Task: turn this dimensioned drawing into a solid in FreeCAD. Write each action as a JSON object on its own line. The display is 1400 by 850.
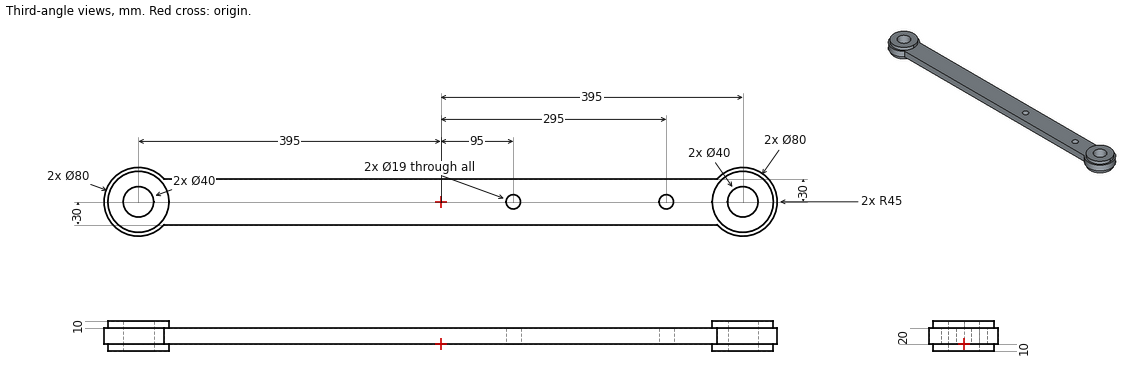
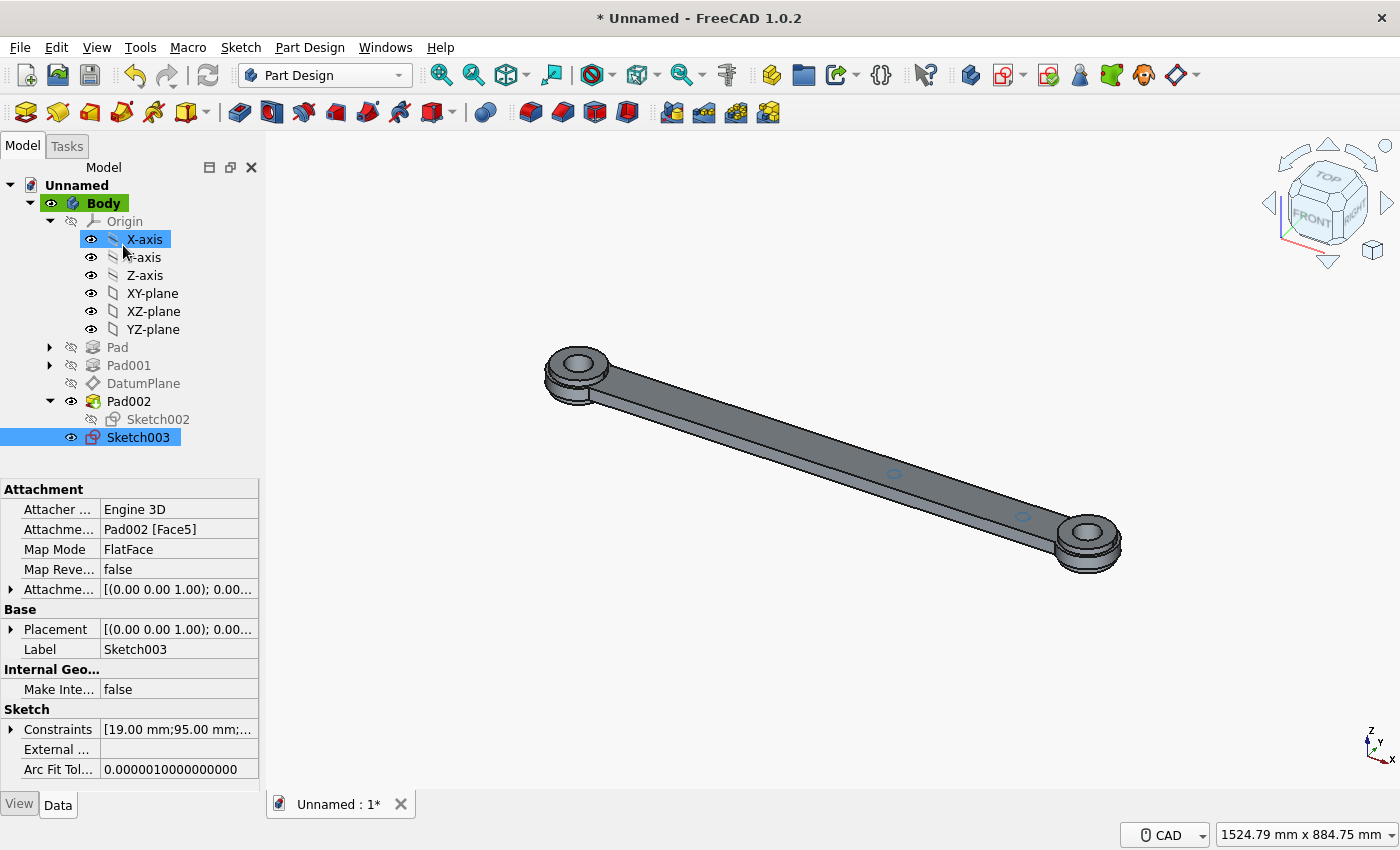
{"action": "left_click", "coordinate": [272, 112]}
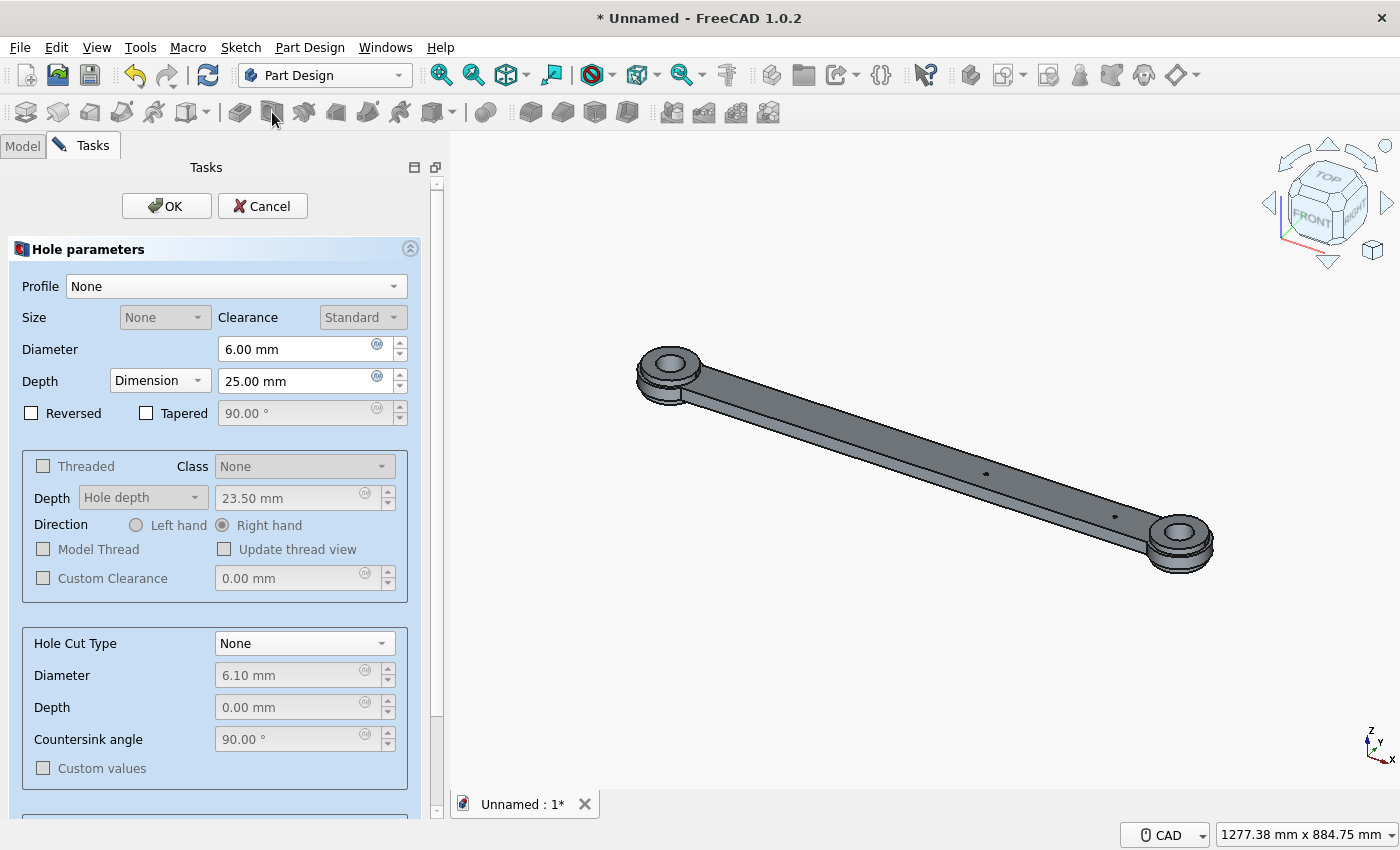
{"action": "triple_click", "coordinate": [305, 349]}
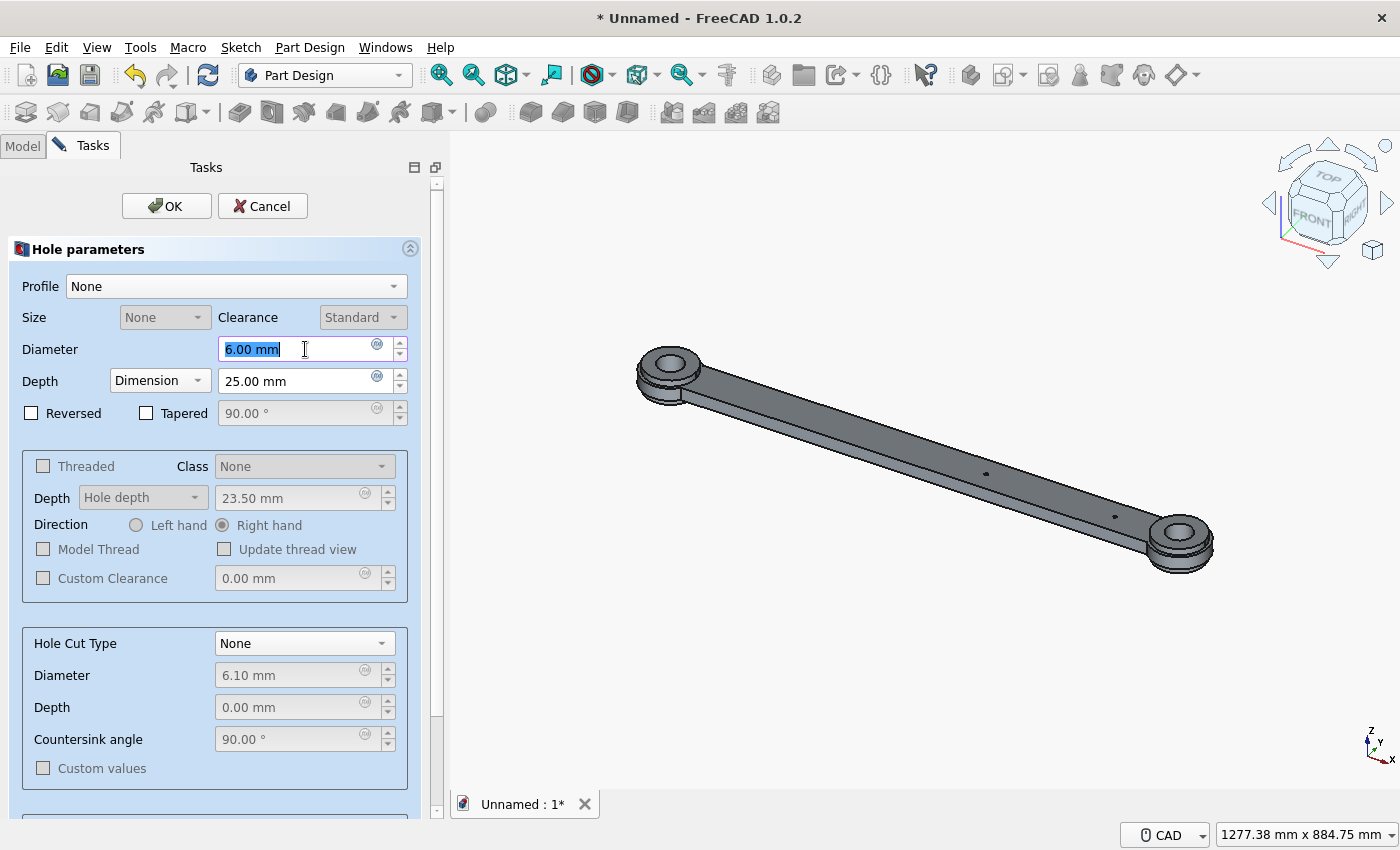
{"action": "type", "text": "19"}
{"action": "key", "text": "Tab"}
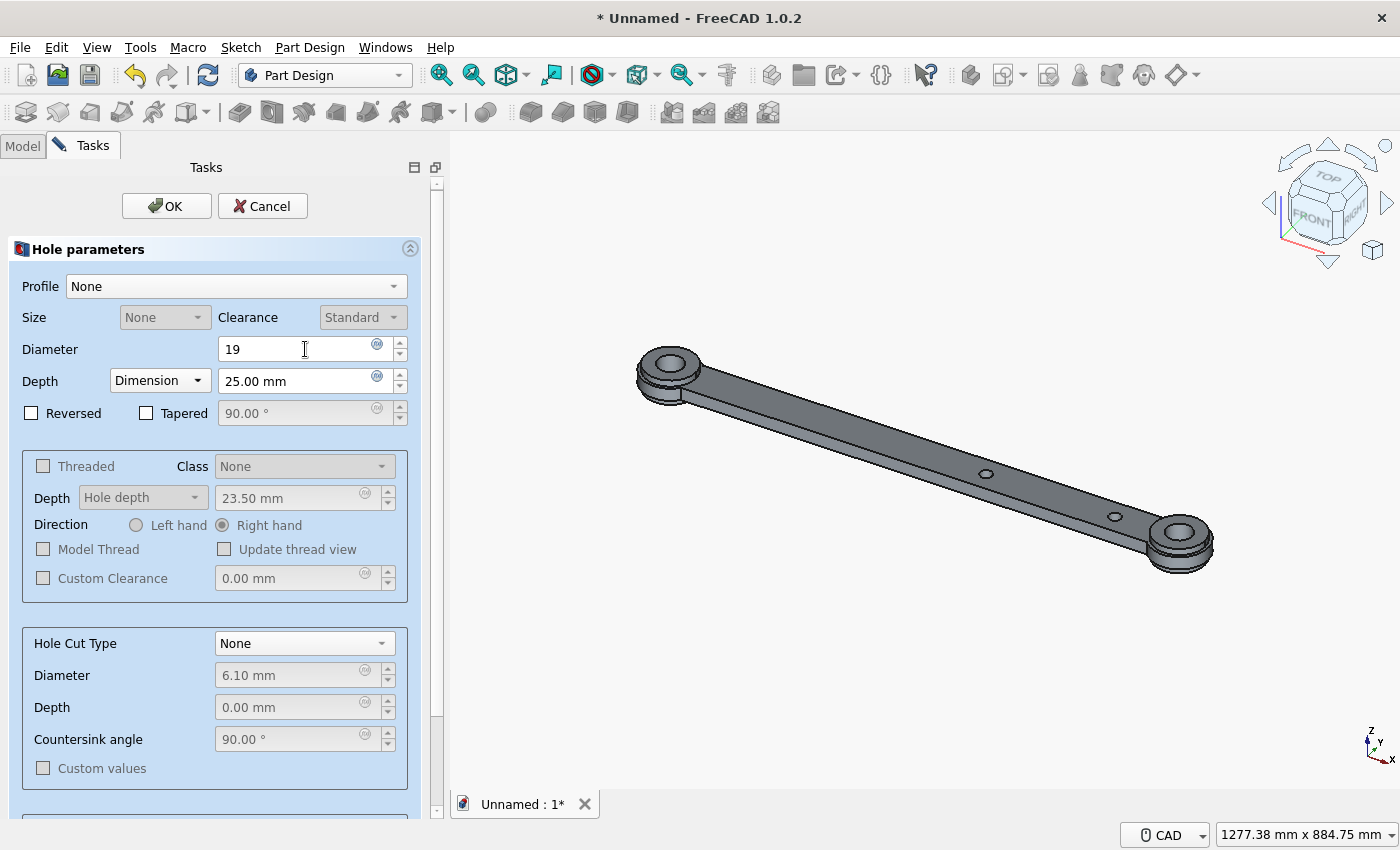
{"action": "left_click", "coordinate": [161, 380]}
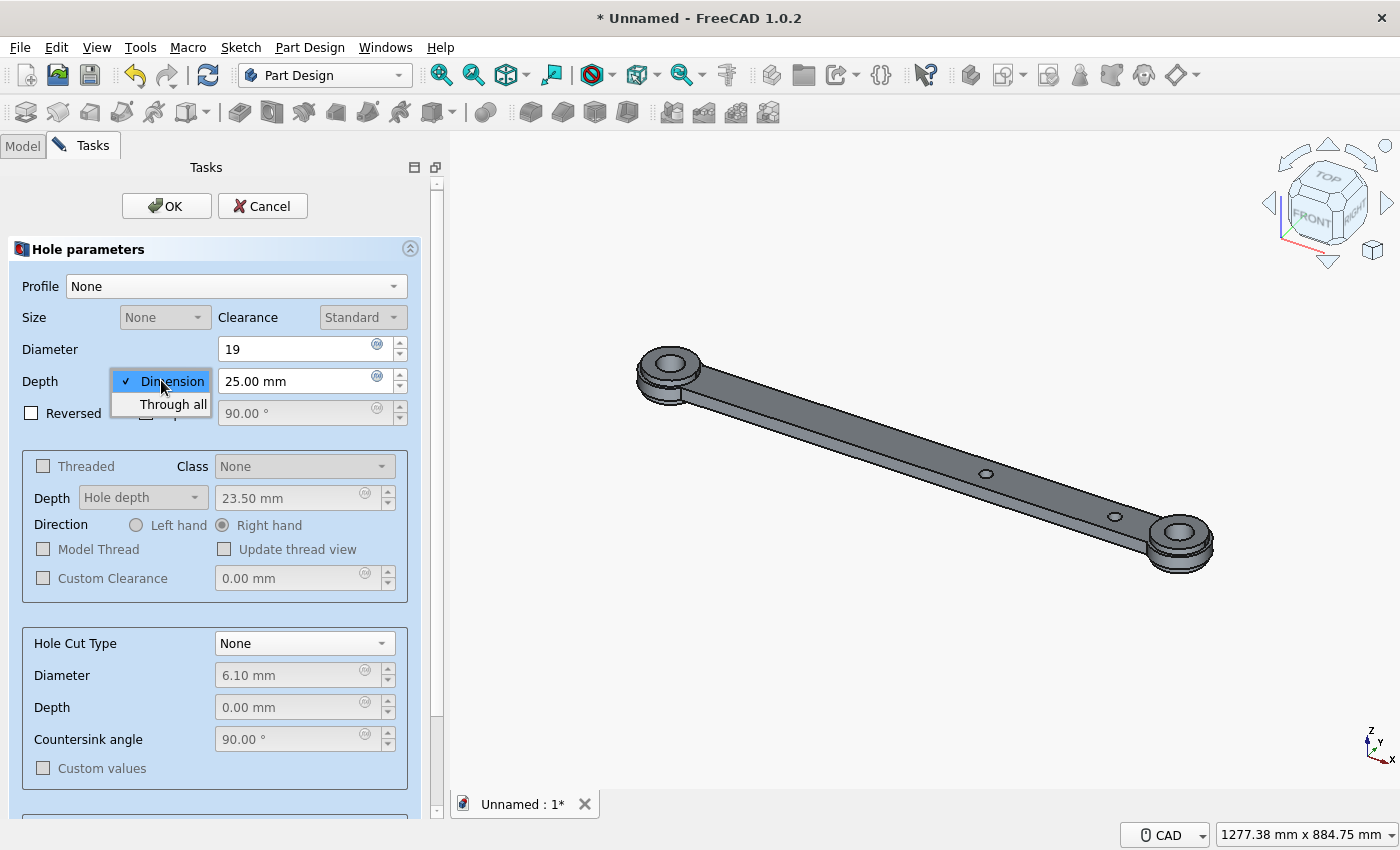
{"action": "left_click", "coordinate": [160, 404]}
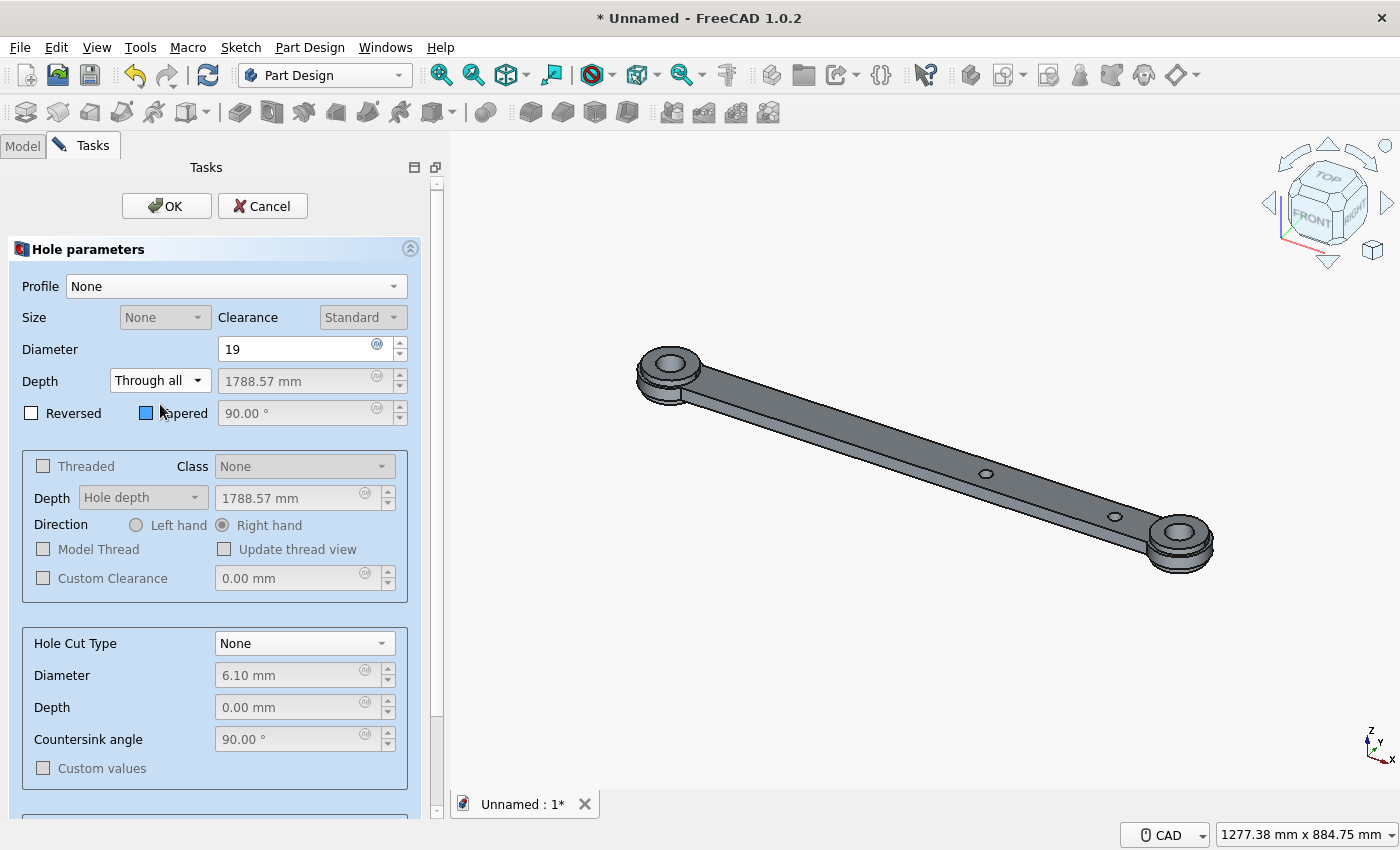
{"action": "left_click", "coordinate": [167, 206]}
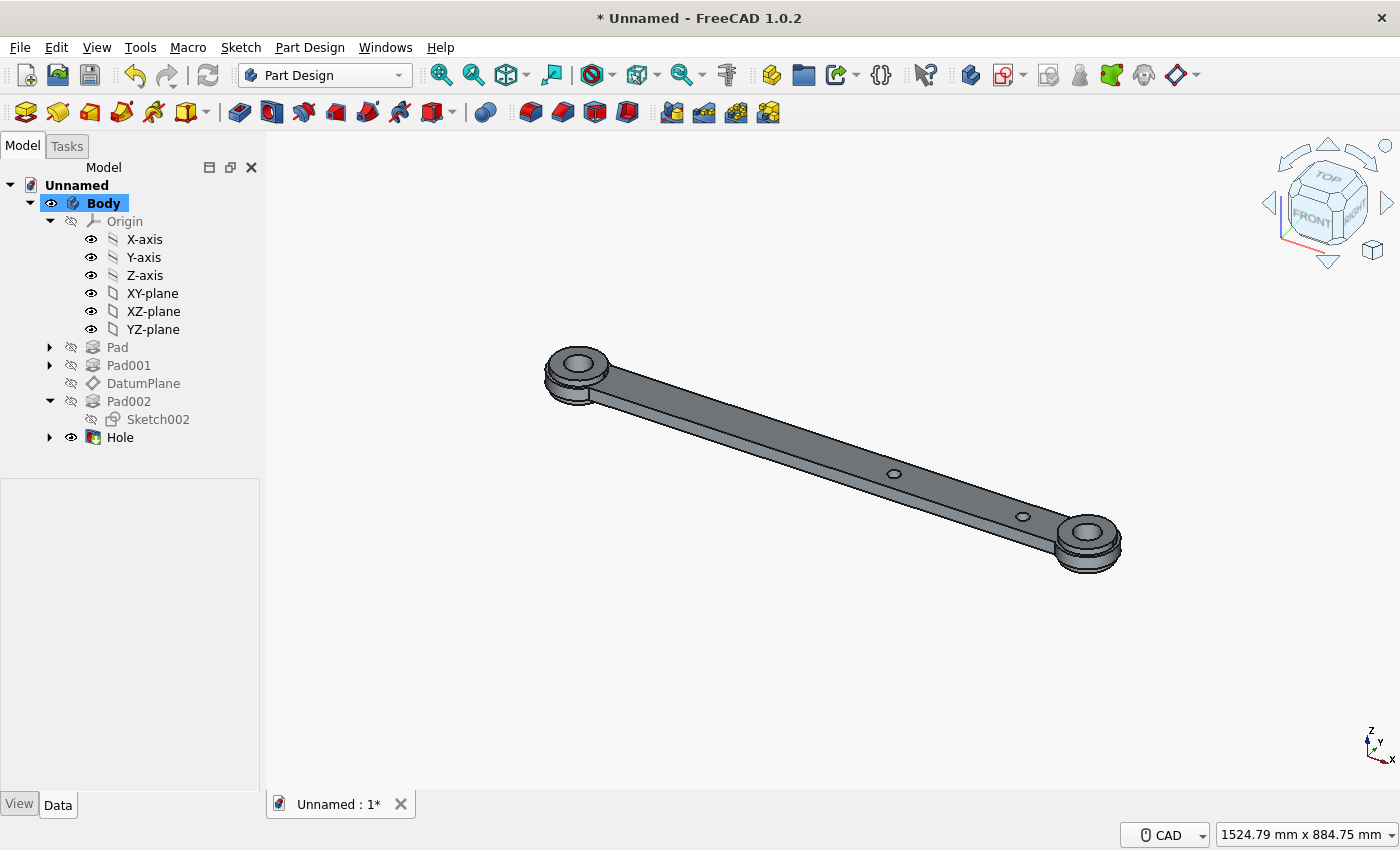
{"action": "key", "text": "0"}